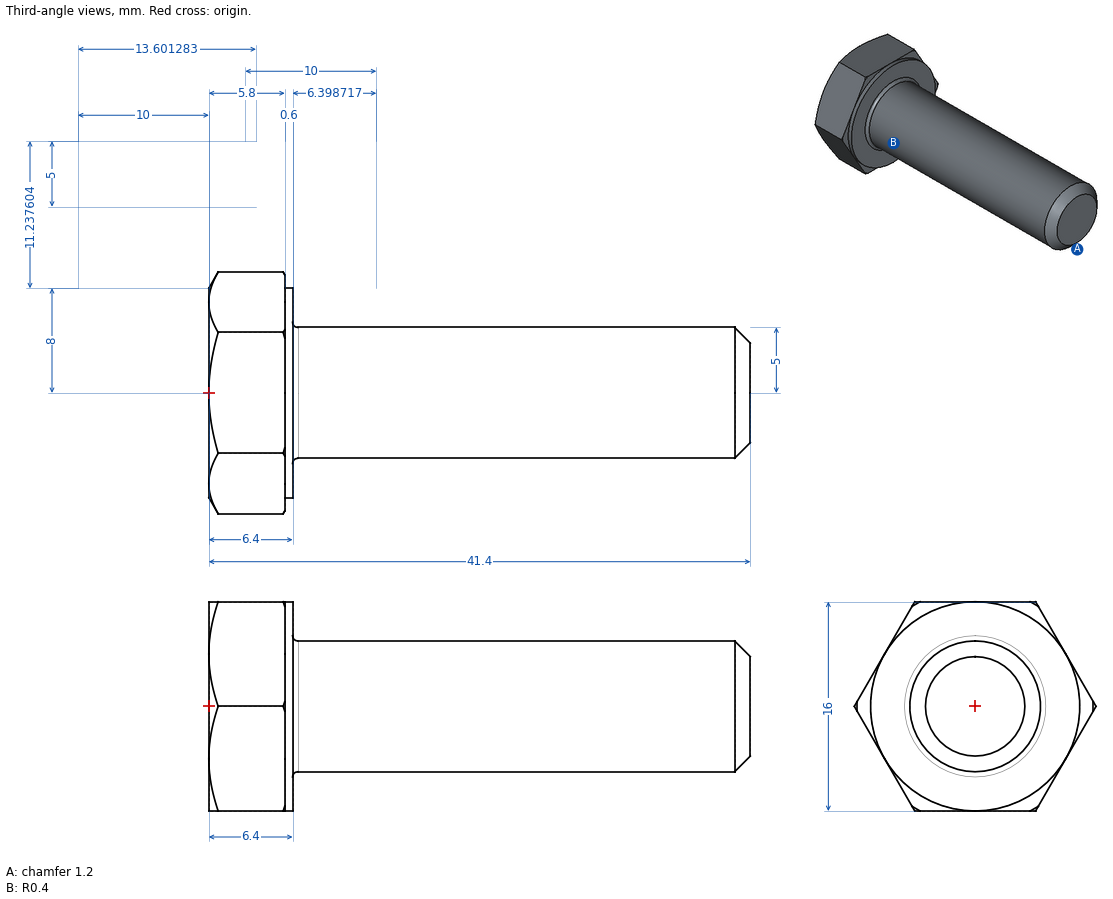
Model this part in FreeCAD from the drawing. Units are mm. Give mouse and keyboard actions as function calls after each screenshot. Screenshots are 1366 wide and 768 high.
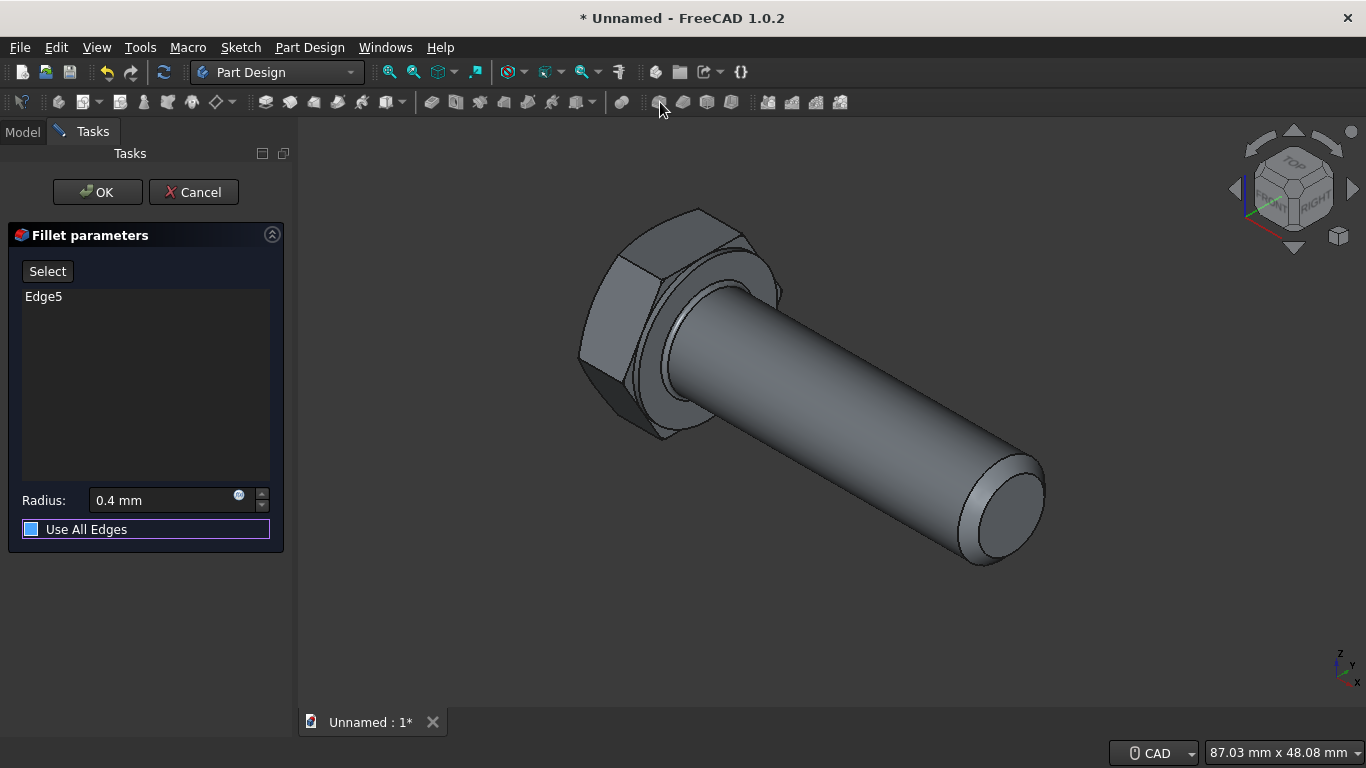
click(98, 192)